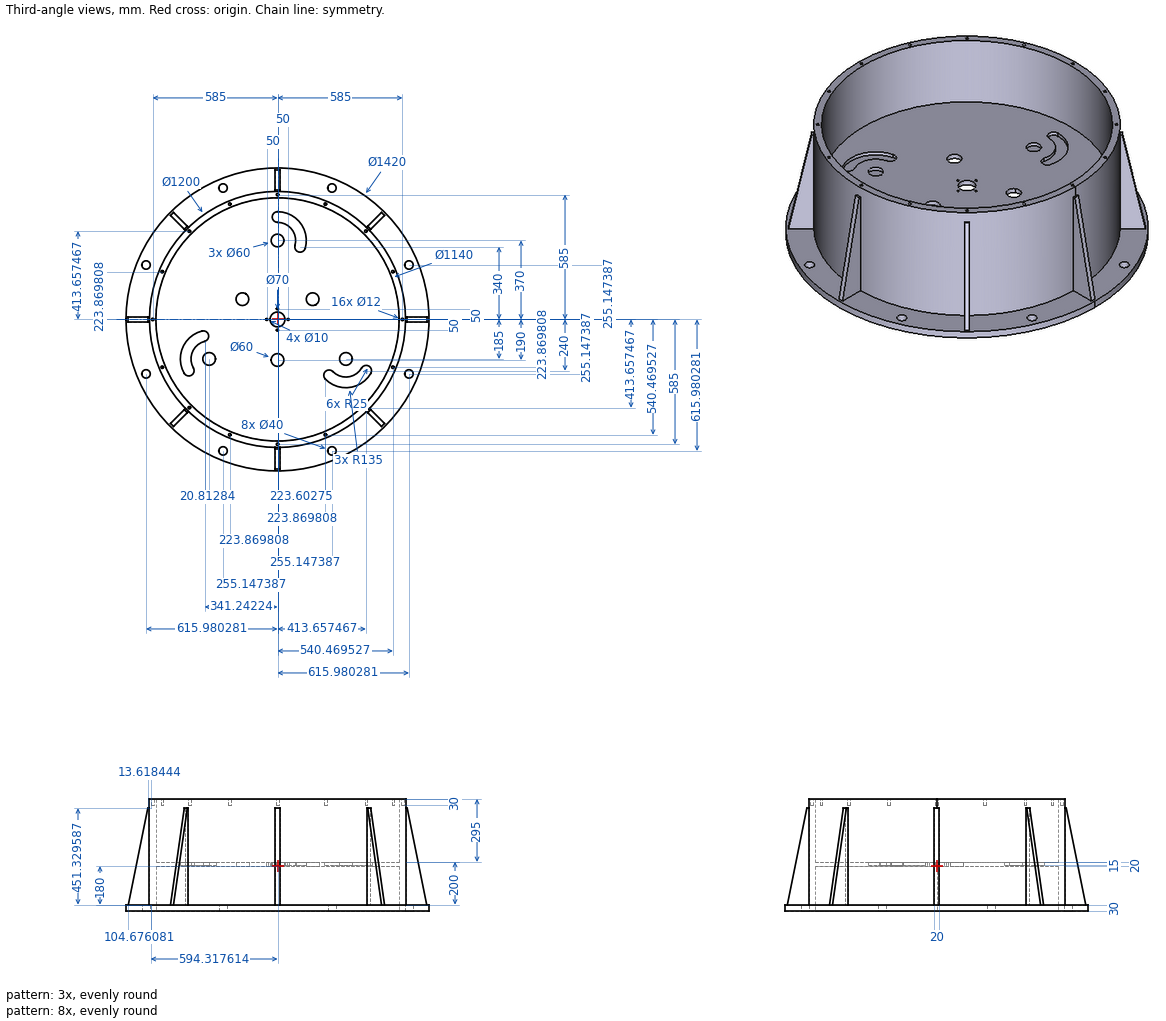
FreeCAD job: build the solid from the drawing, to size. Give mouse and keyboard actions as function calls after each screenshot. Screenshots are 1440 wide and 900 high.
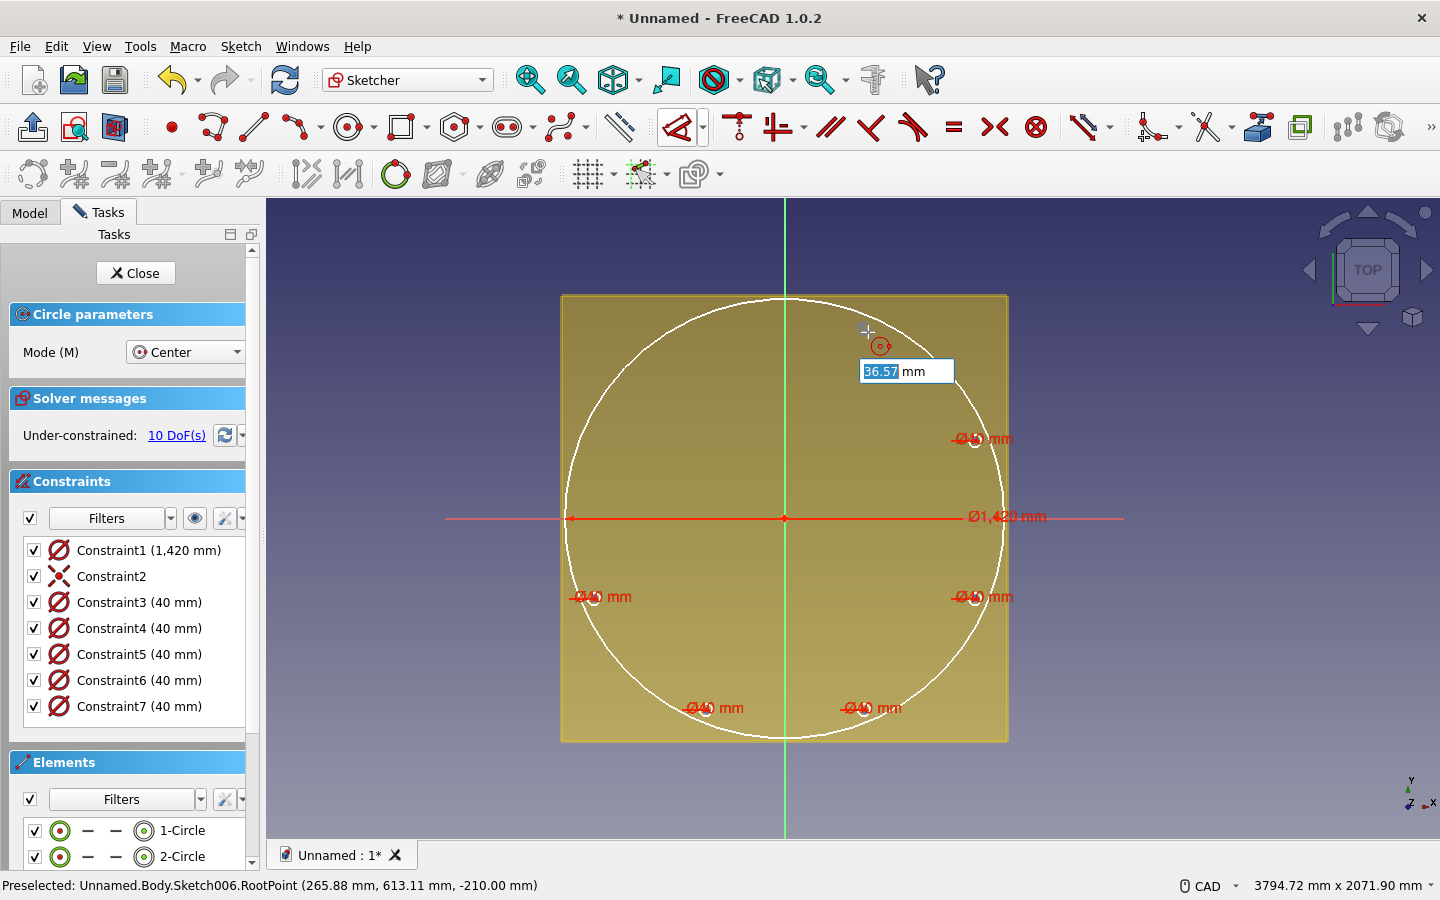
text(40)
key(Return)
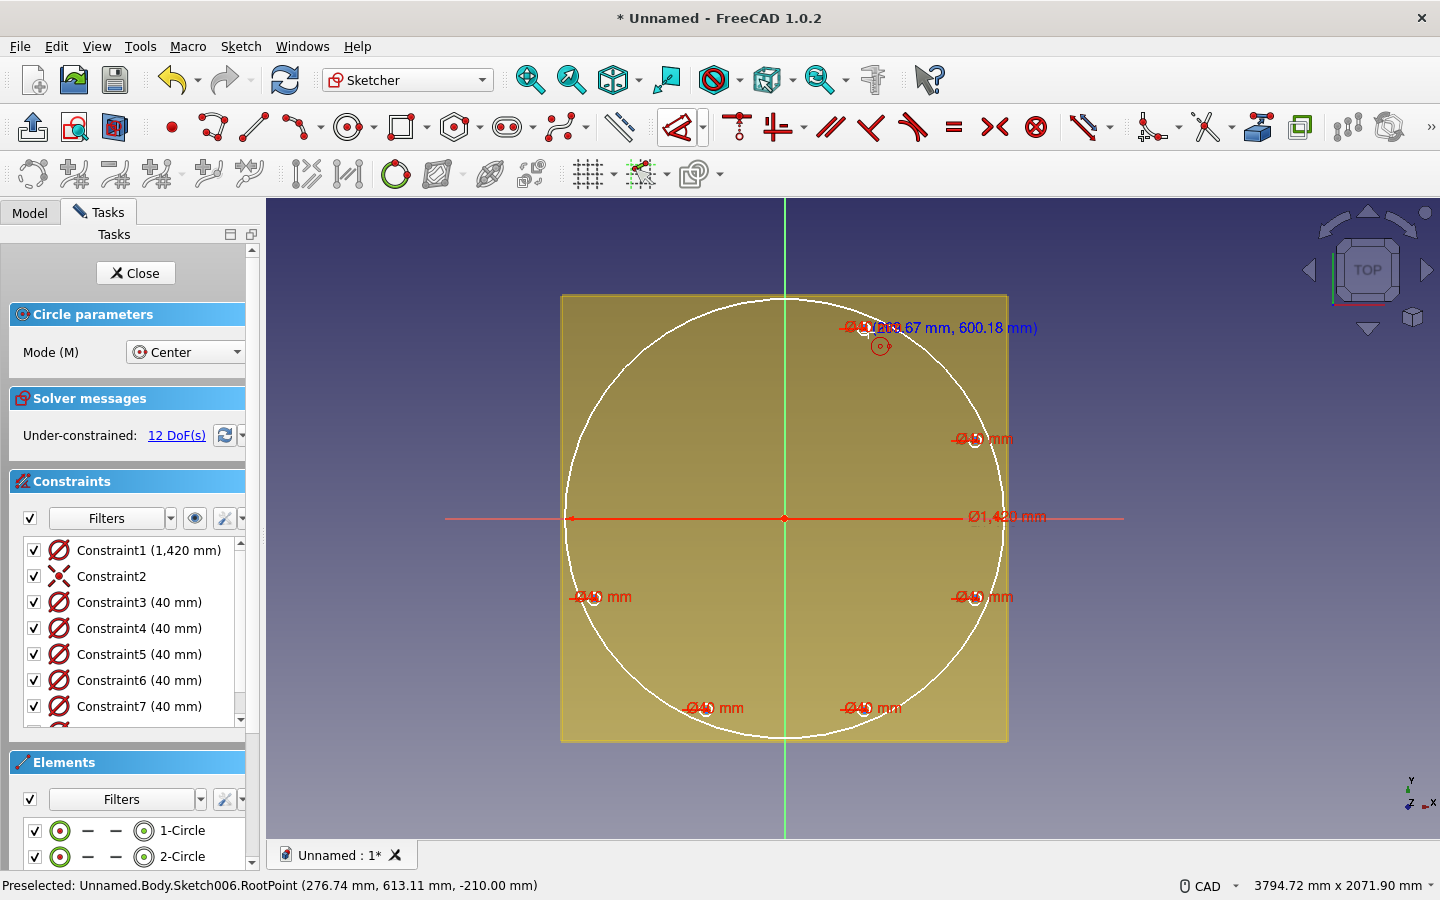
click(785, 519)
move(909, 394)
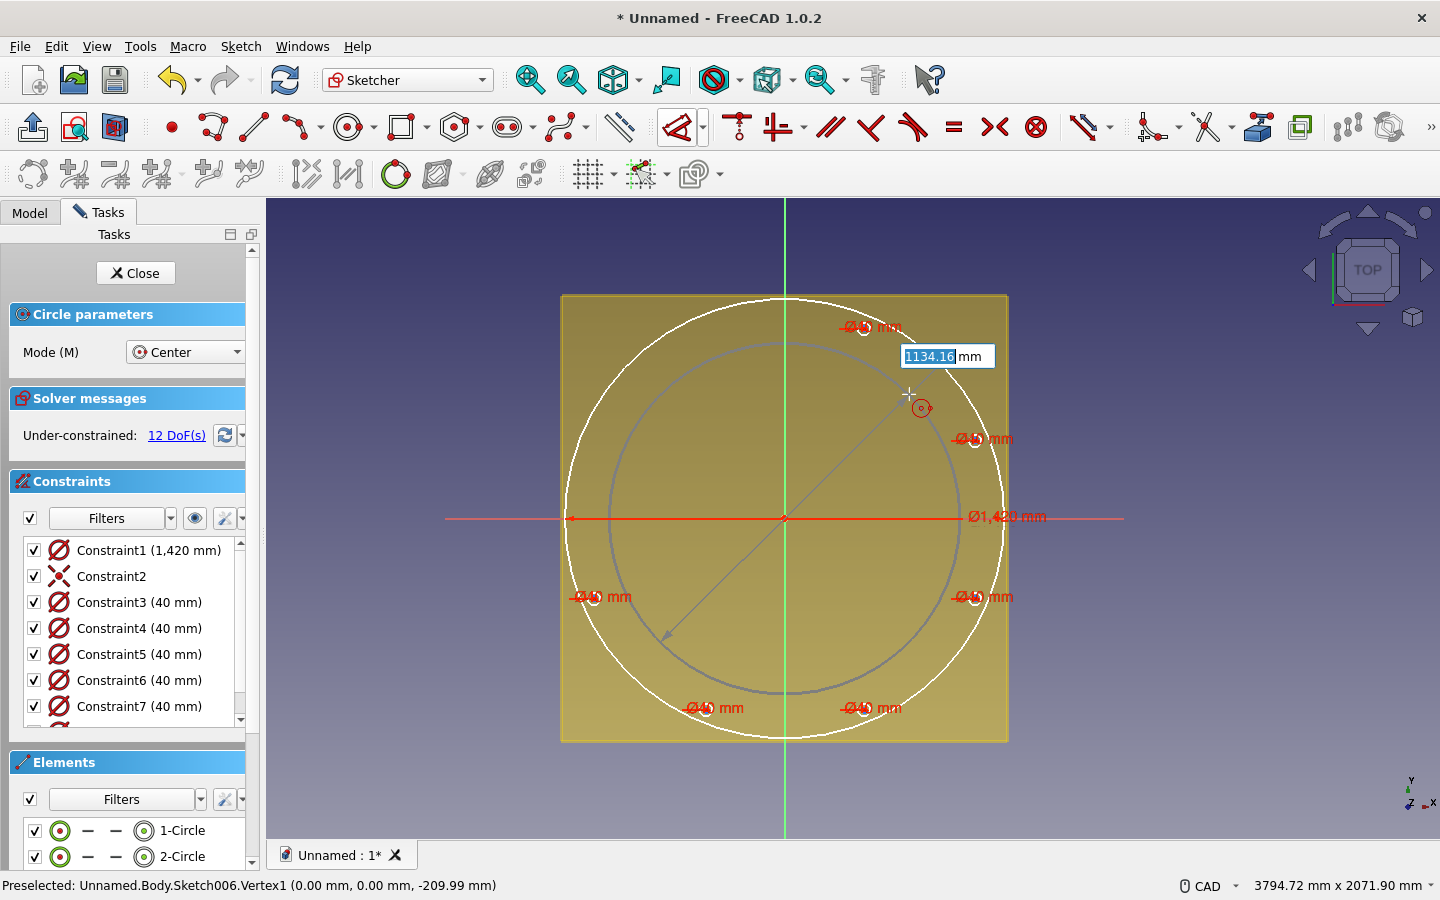
text(1140)
key(Return)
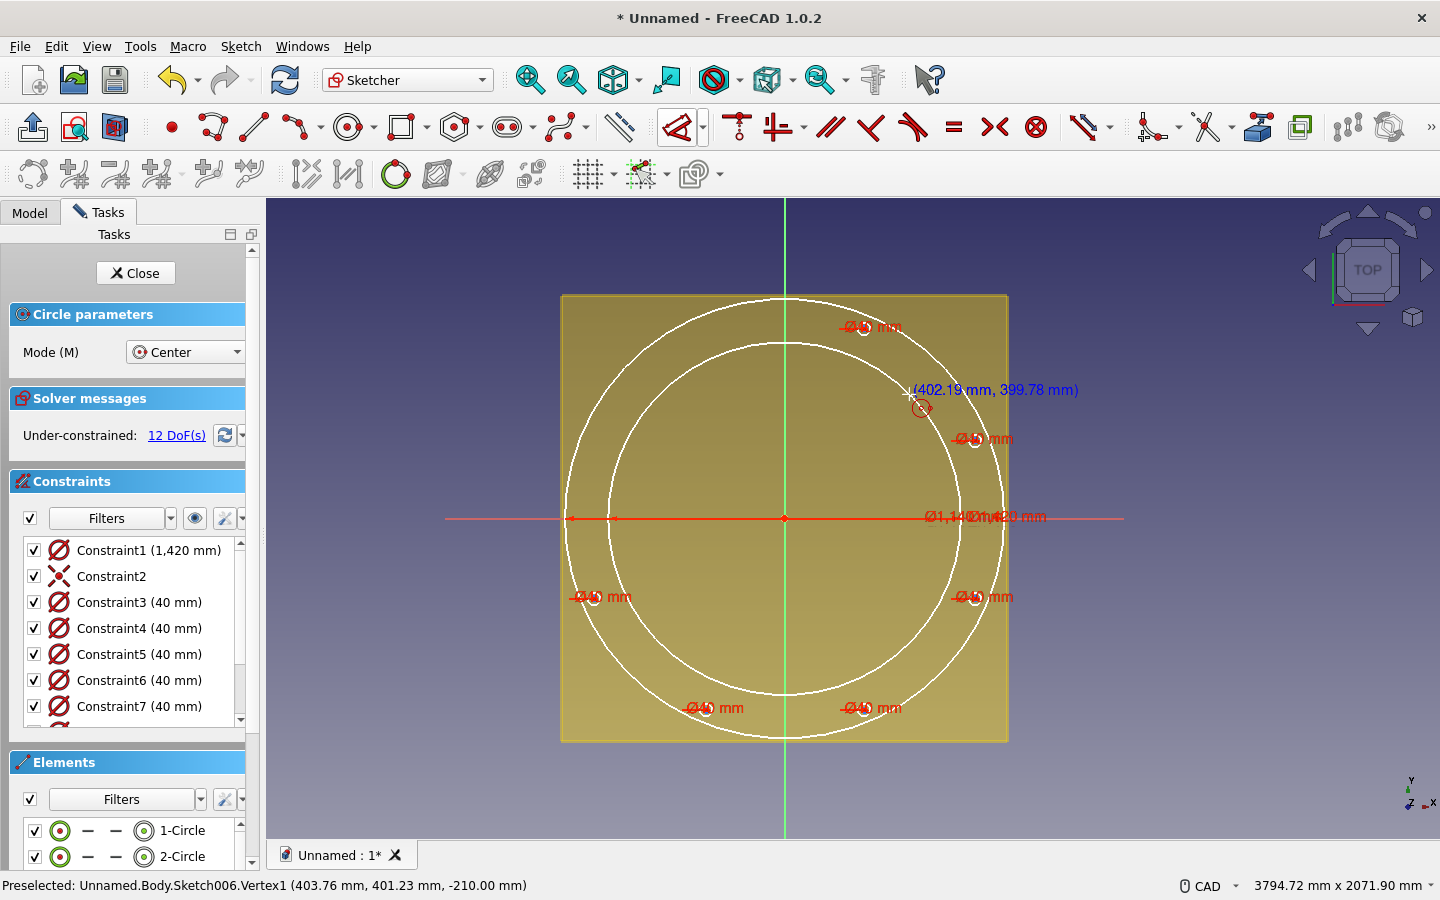
scroll(594, 440, up, 7)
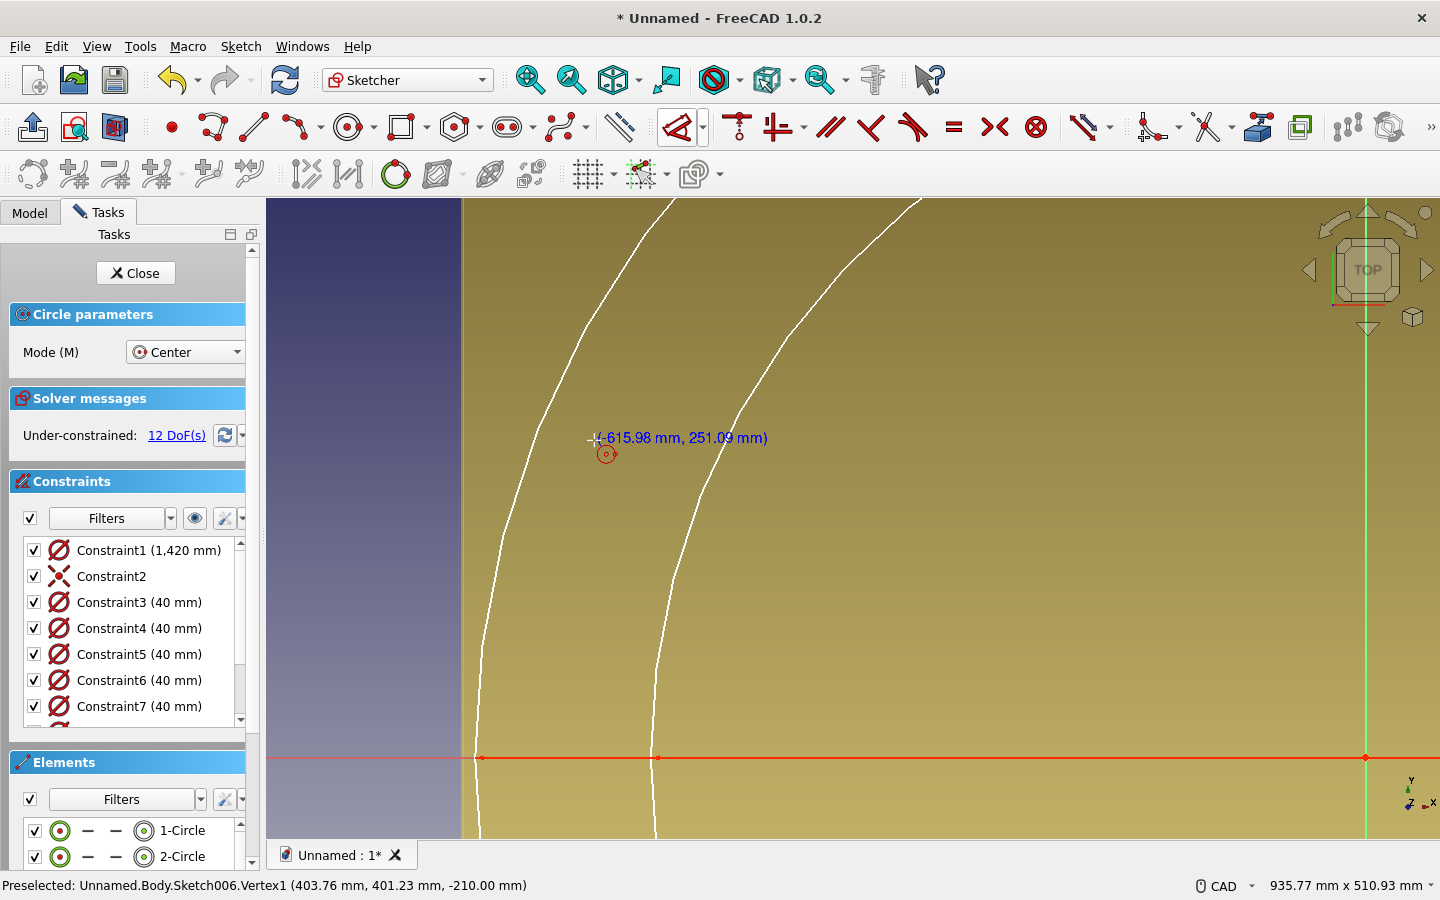
scroll(594, 440, down, 7)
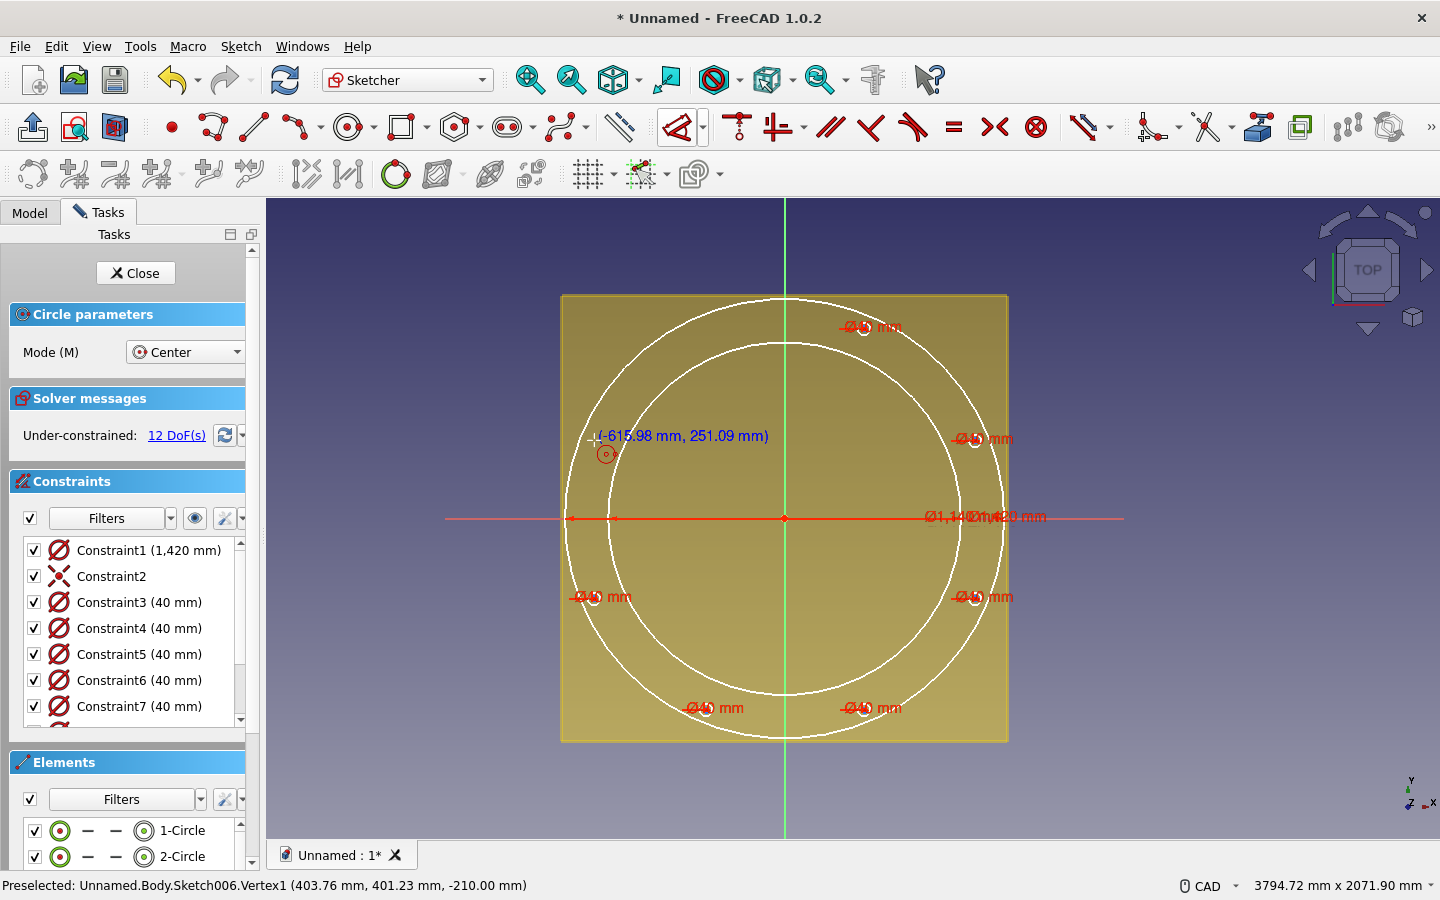
click(594, 440)
move(598, 435)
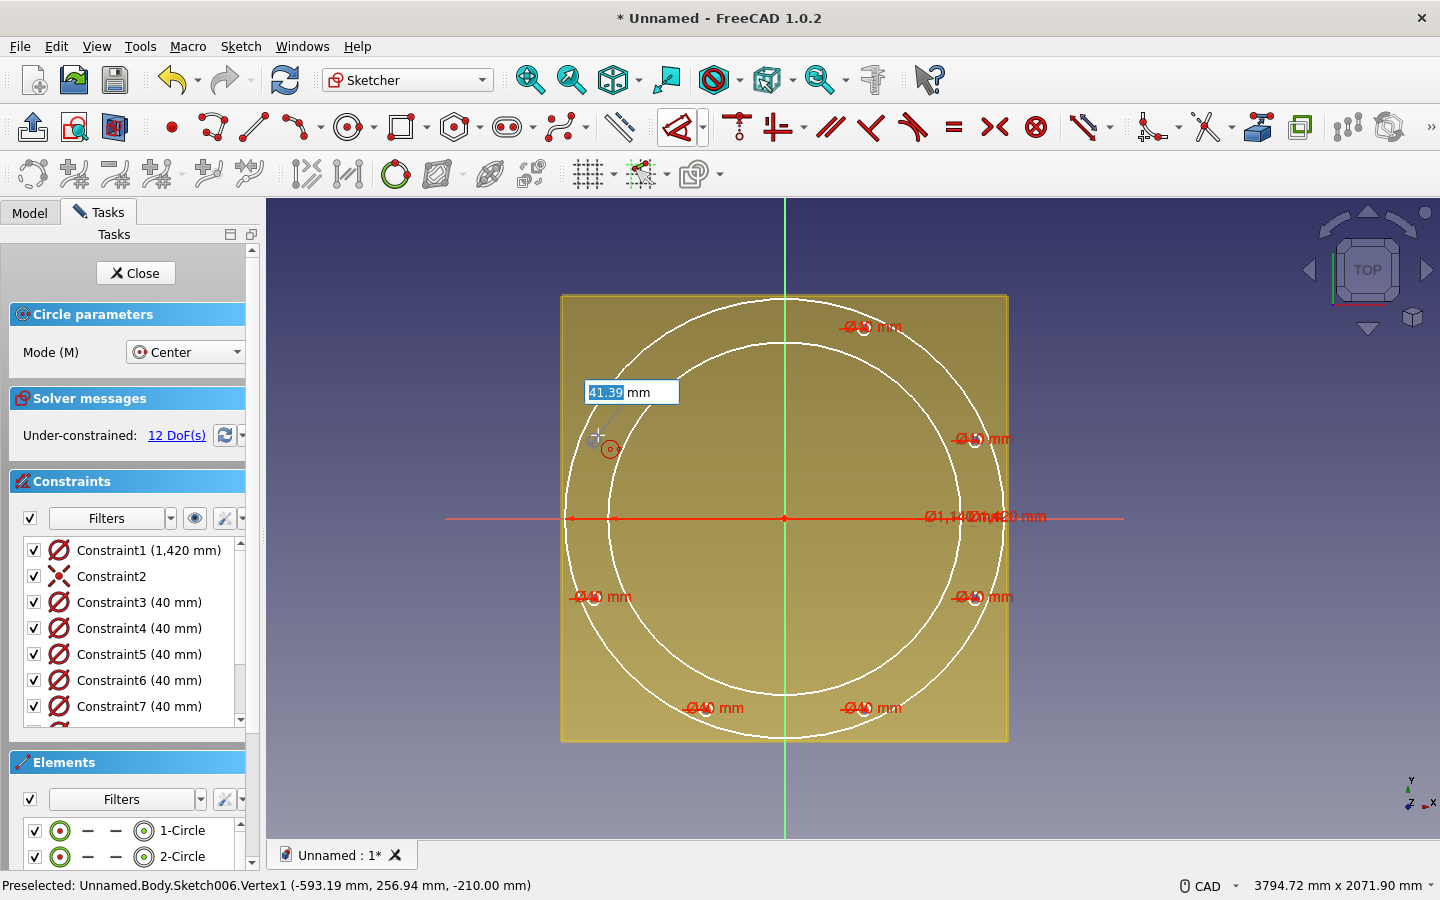
text(40)
key(Return)